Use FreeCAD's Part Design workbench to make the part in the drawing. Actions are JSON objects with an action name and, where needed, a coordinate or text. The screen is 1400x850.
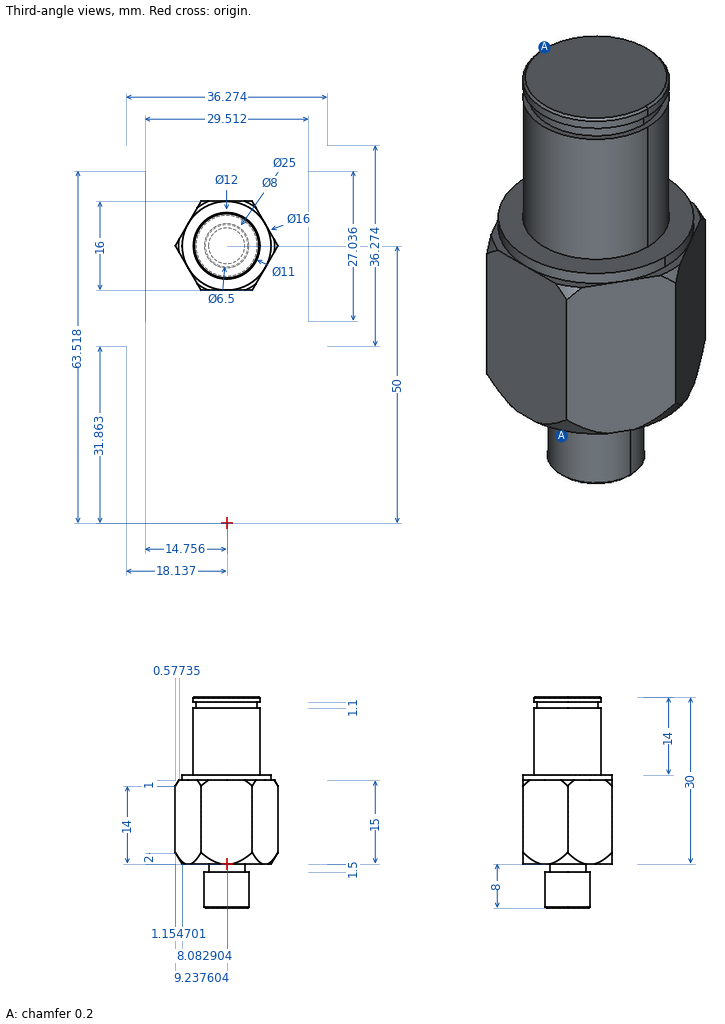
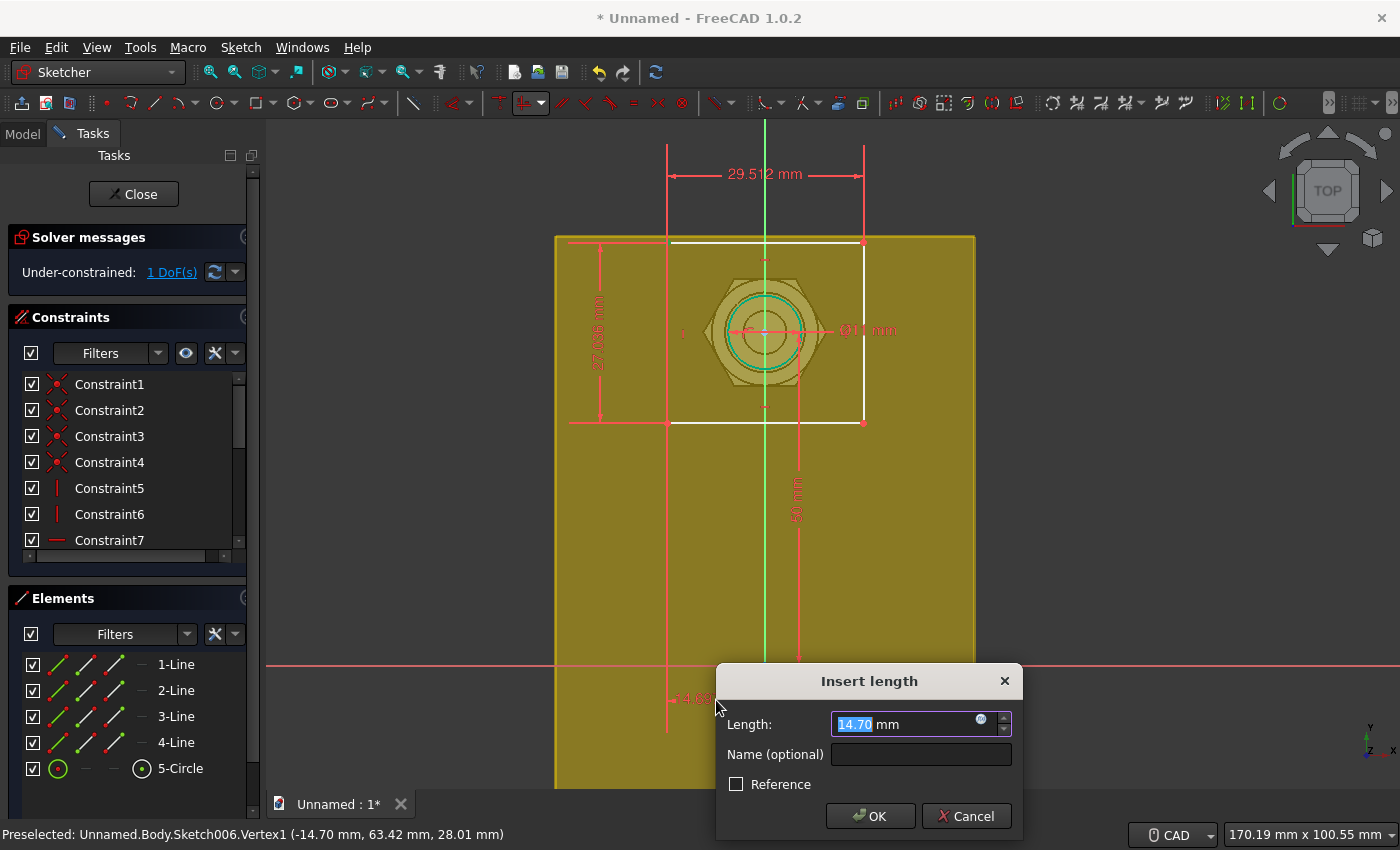
{"action": "type", "text": "14.756"}
{"action": "key", "text": "Return"}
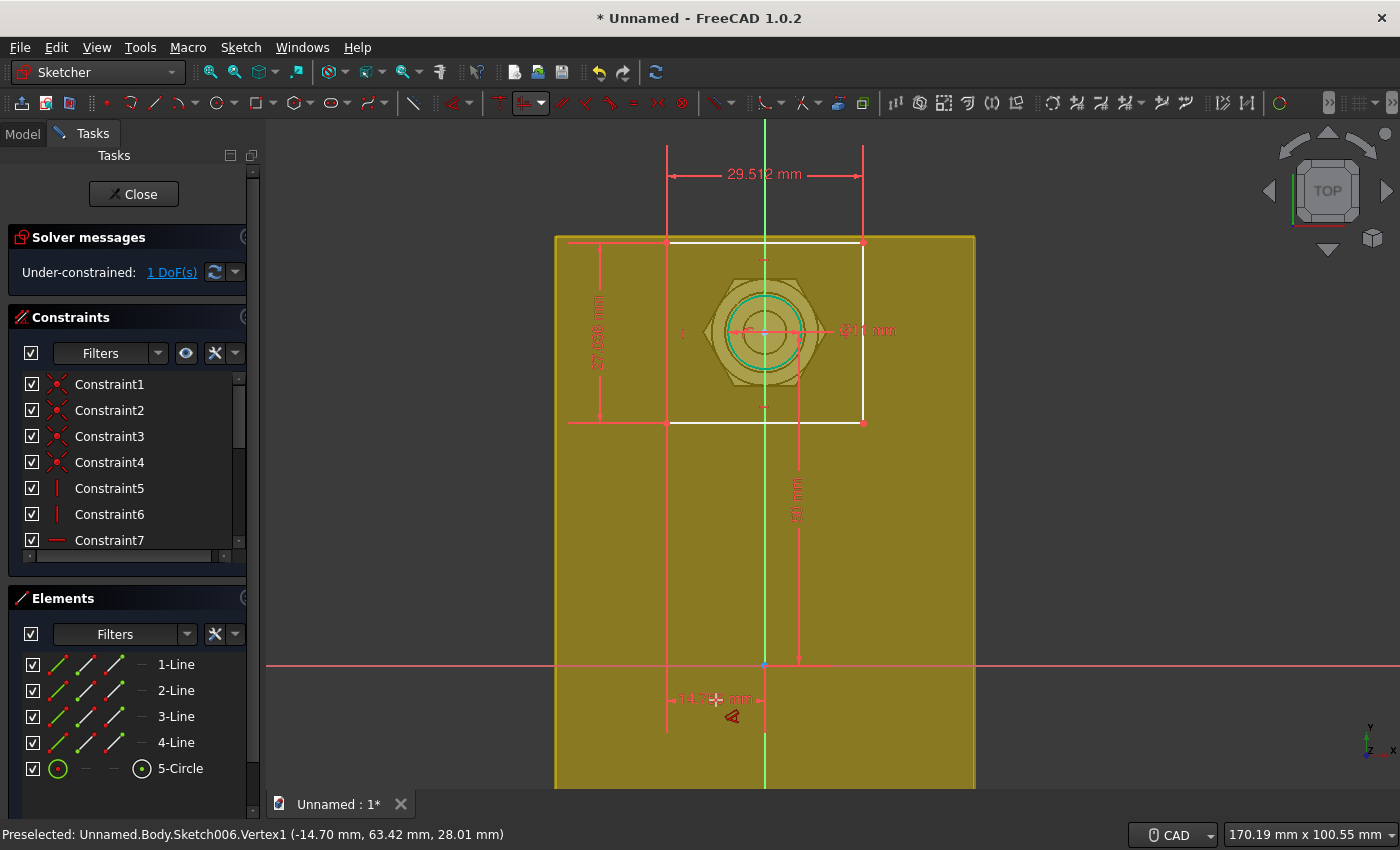
{"action": "left_click", "coordinate": [667, 243]}
{"action": "left_click", "coordinate": [633, 454]}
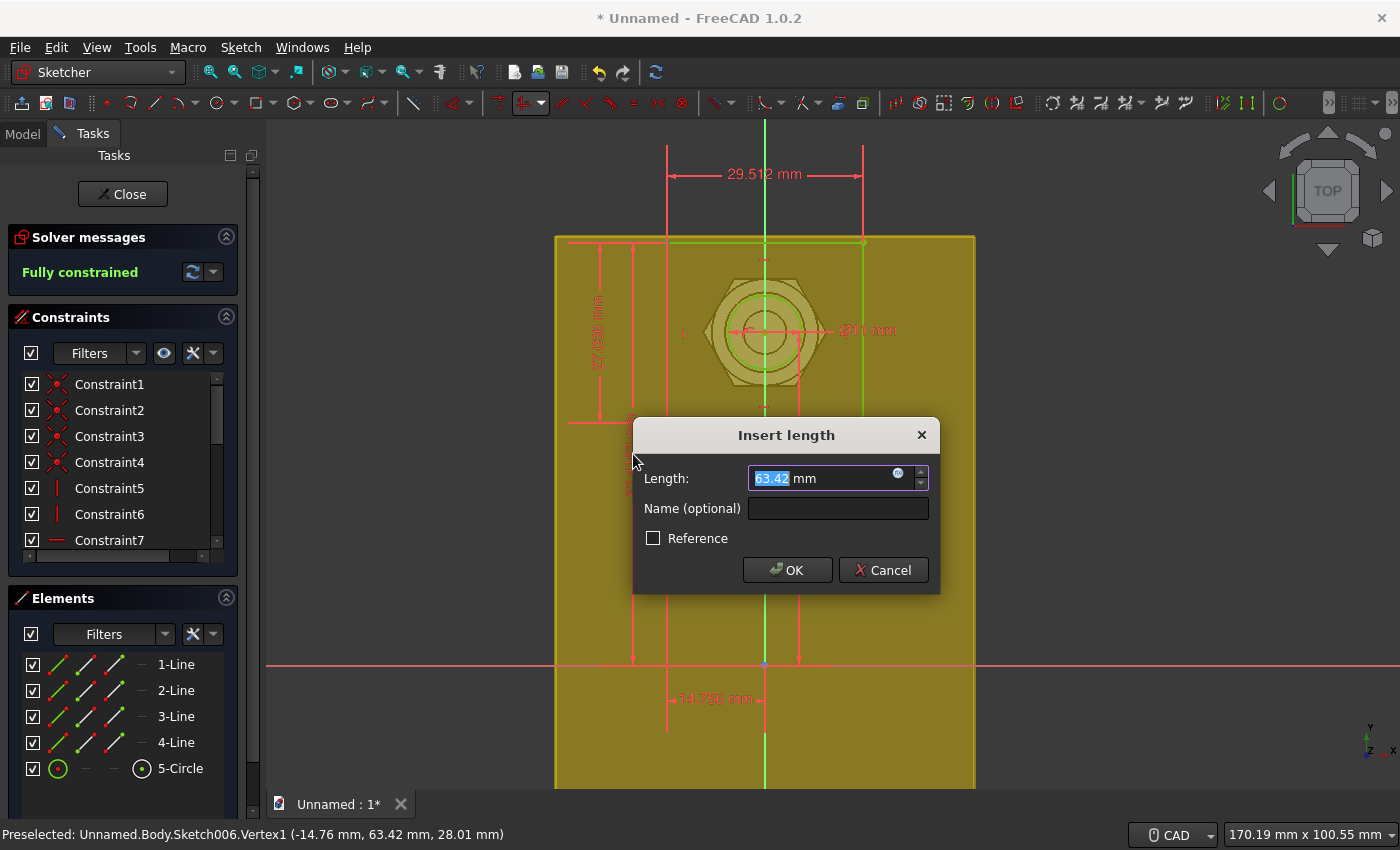
{"action": "type", "text": "63.518"}
{"action": "key", "text": "Return"}
{"action": "key", "text": "Escape"}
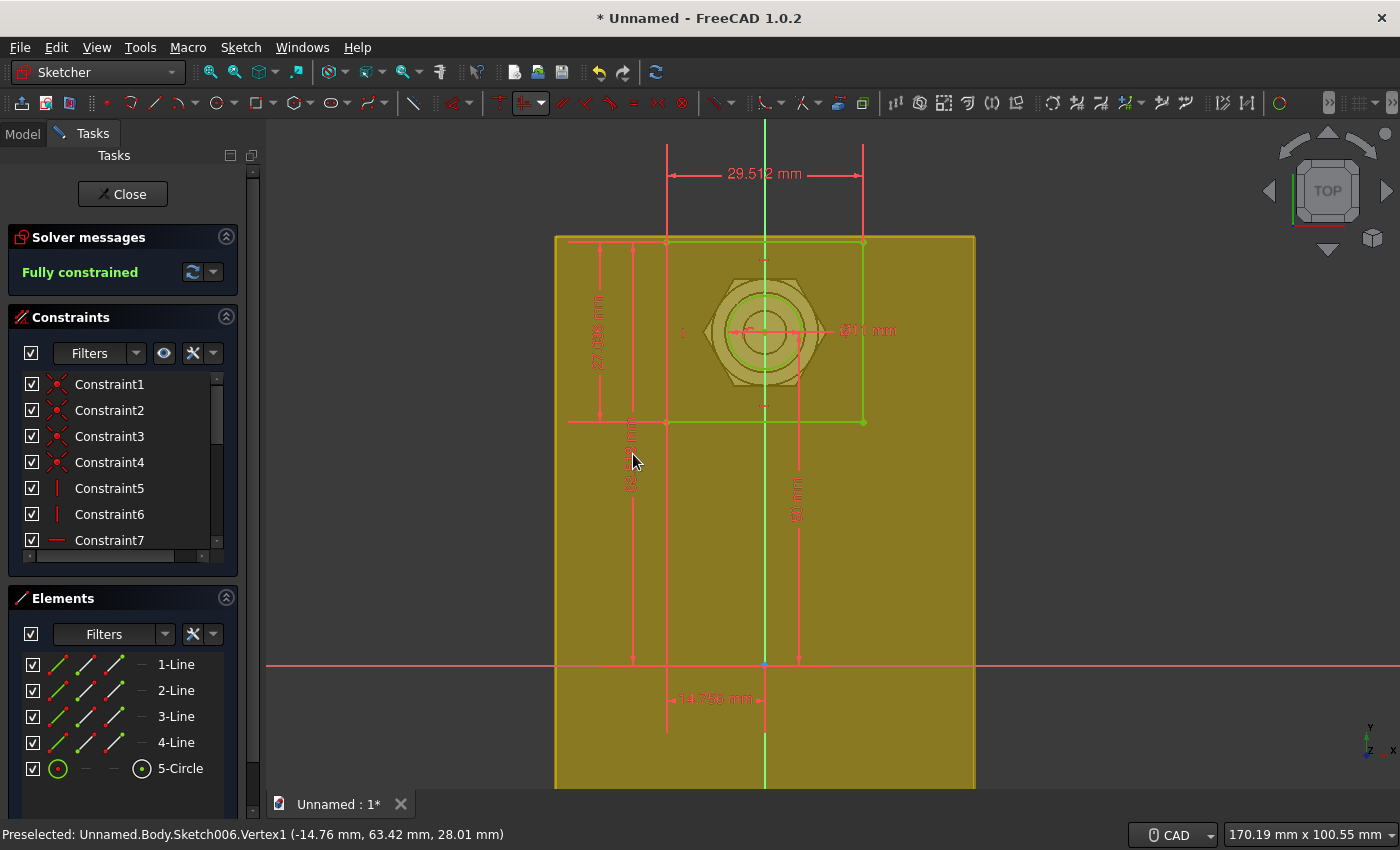
{"action": "left_click", "coordinate": [123, 194]}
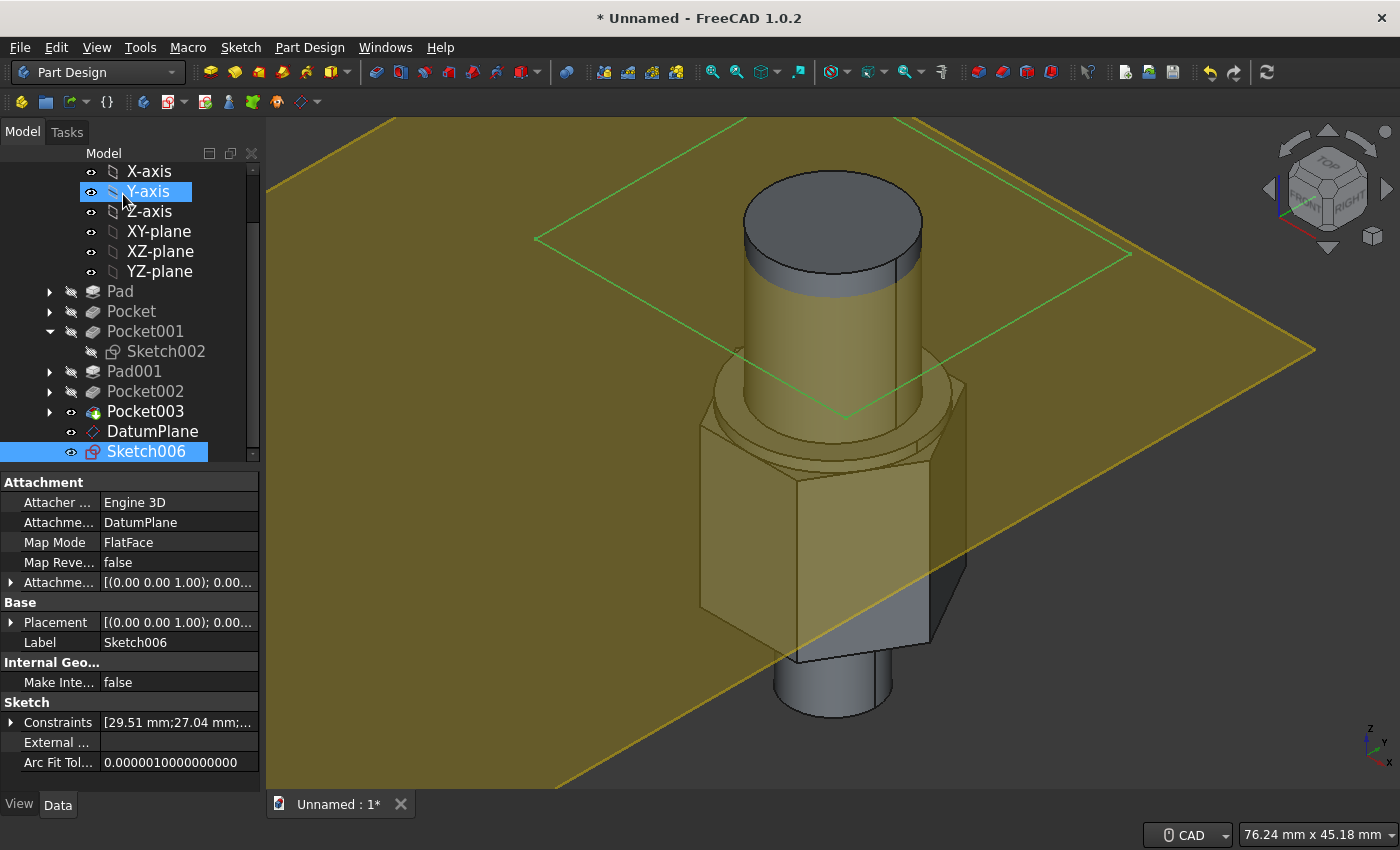
{"action": "left_click", "coordinate": [378, 72]}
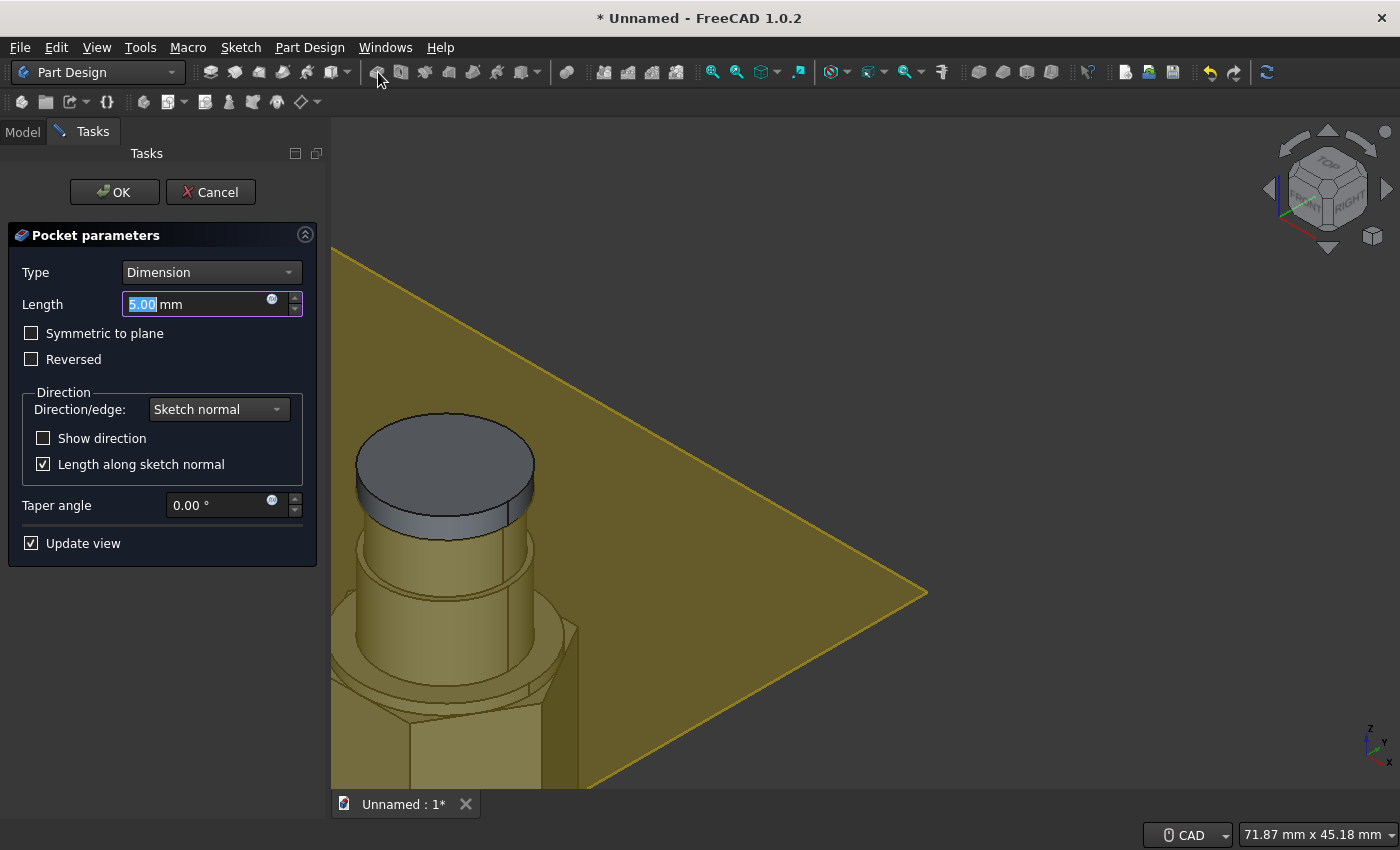
{"action": "type", "text": "1.1"}
{"action": "key", "text": "Tab"}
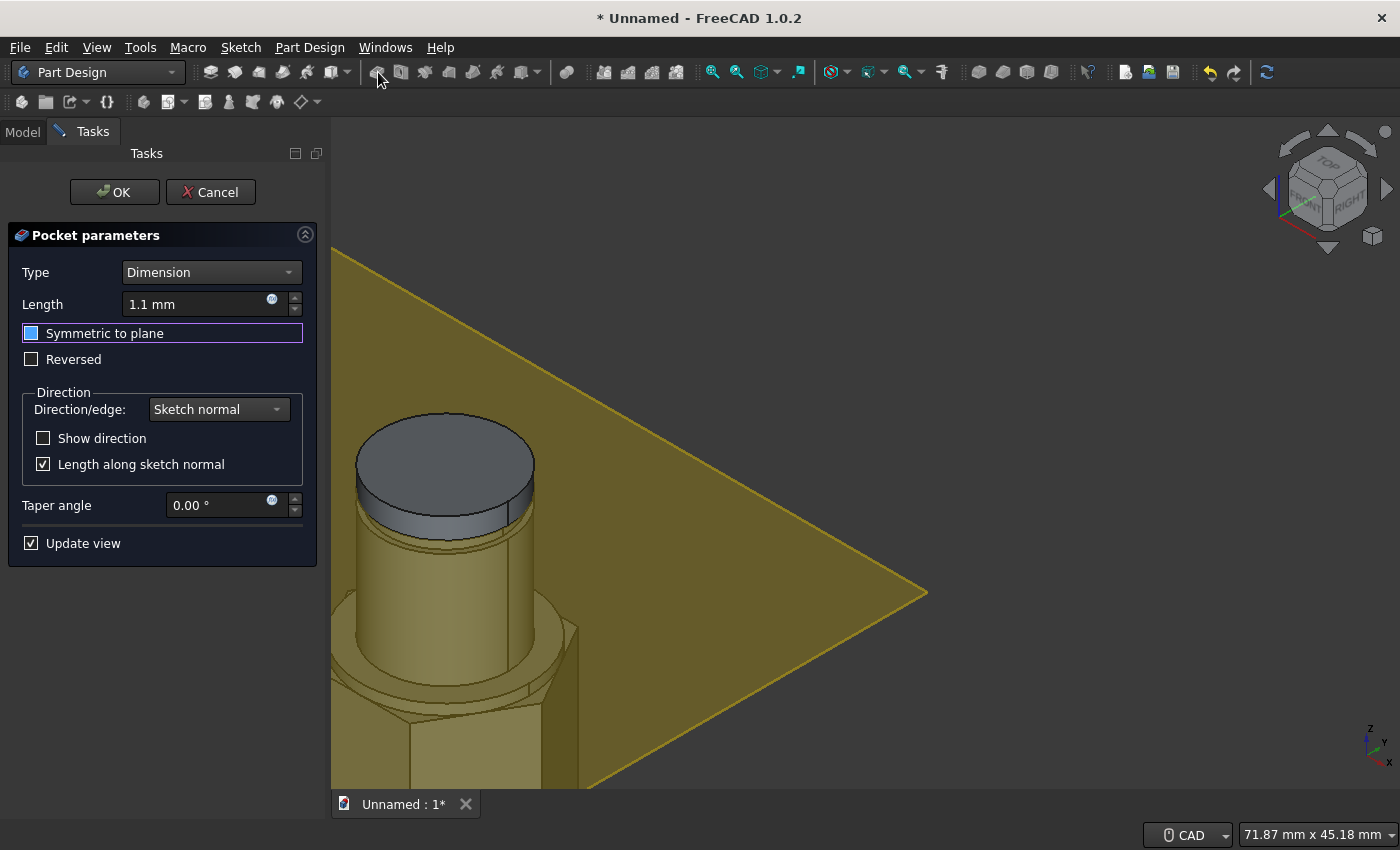
{"action": "left_click", "coordinate": [30, 359]}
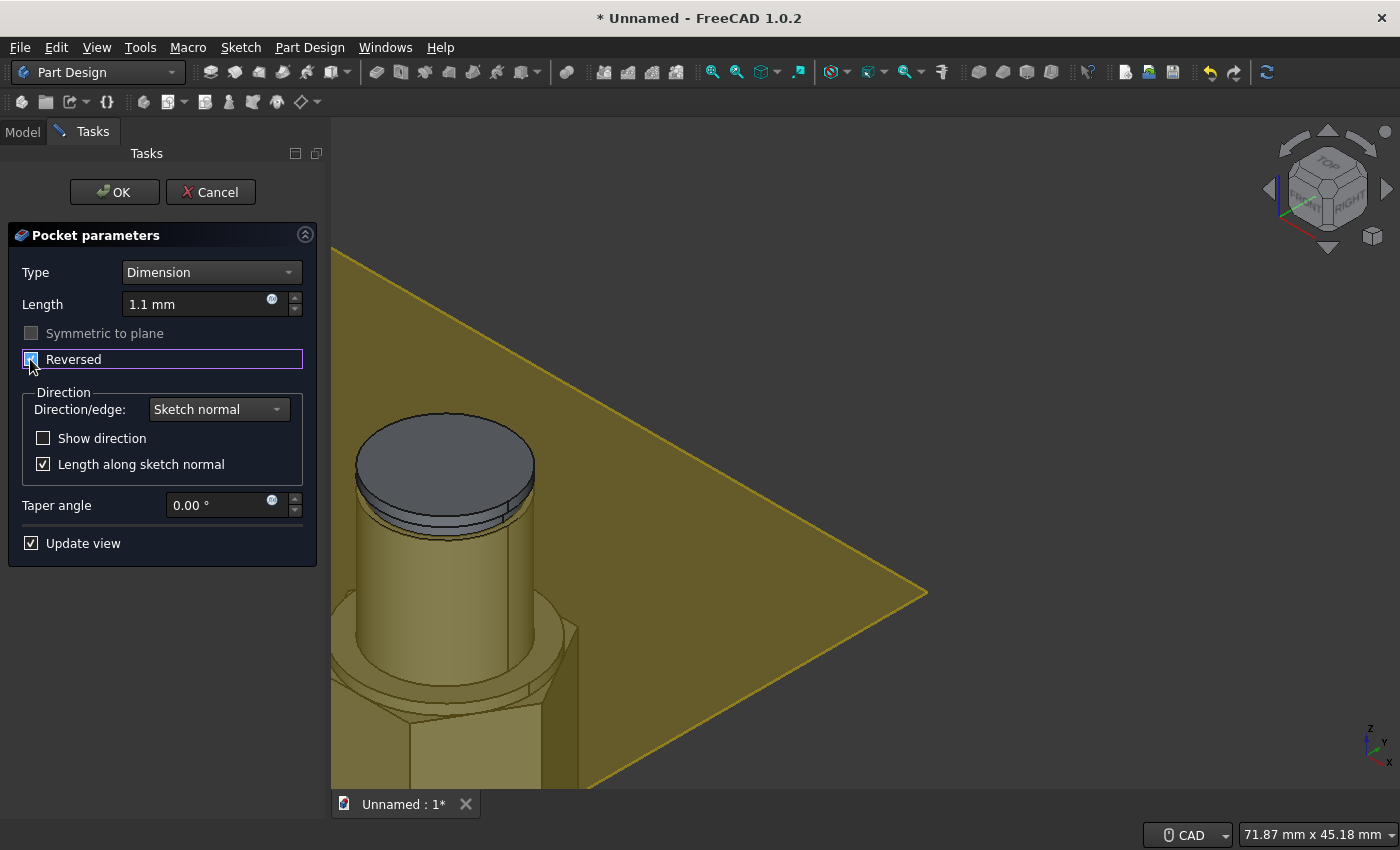
{"action": "left_click", "coordinate": [115, 192]}